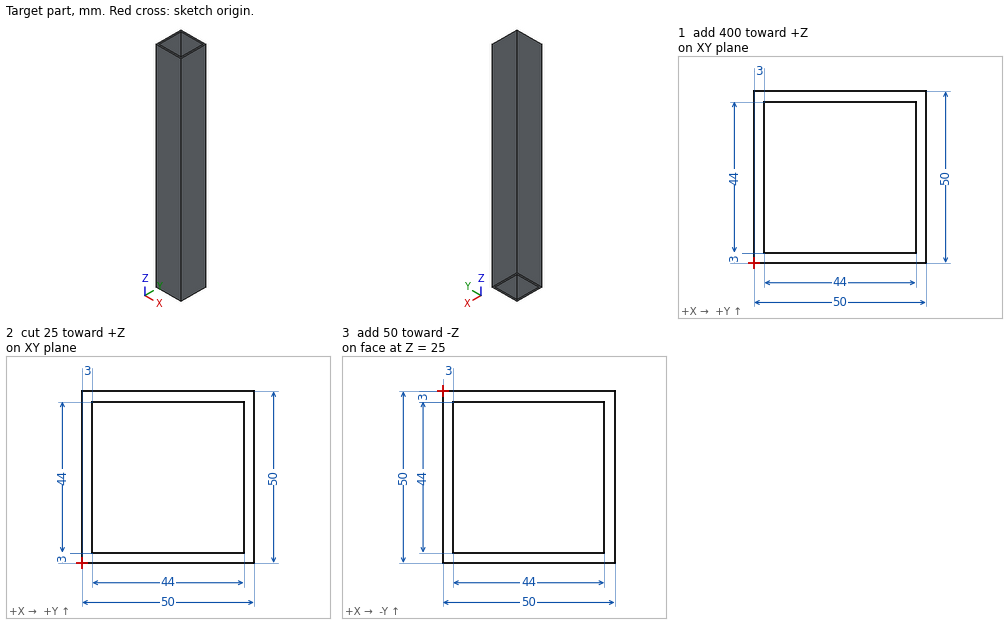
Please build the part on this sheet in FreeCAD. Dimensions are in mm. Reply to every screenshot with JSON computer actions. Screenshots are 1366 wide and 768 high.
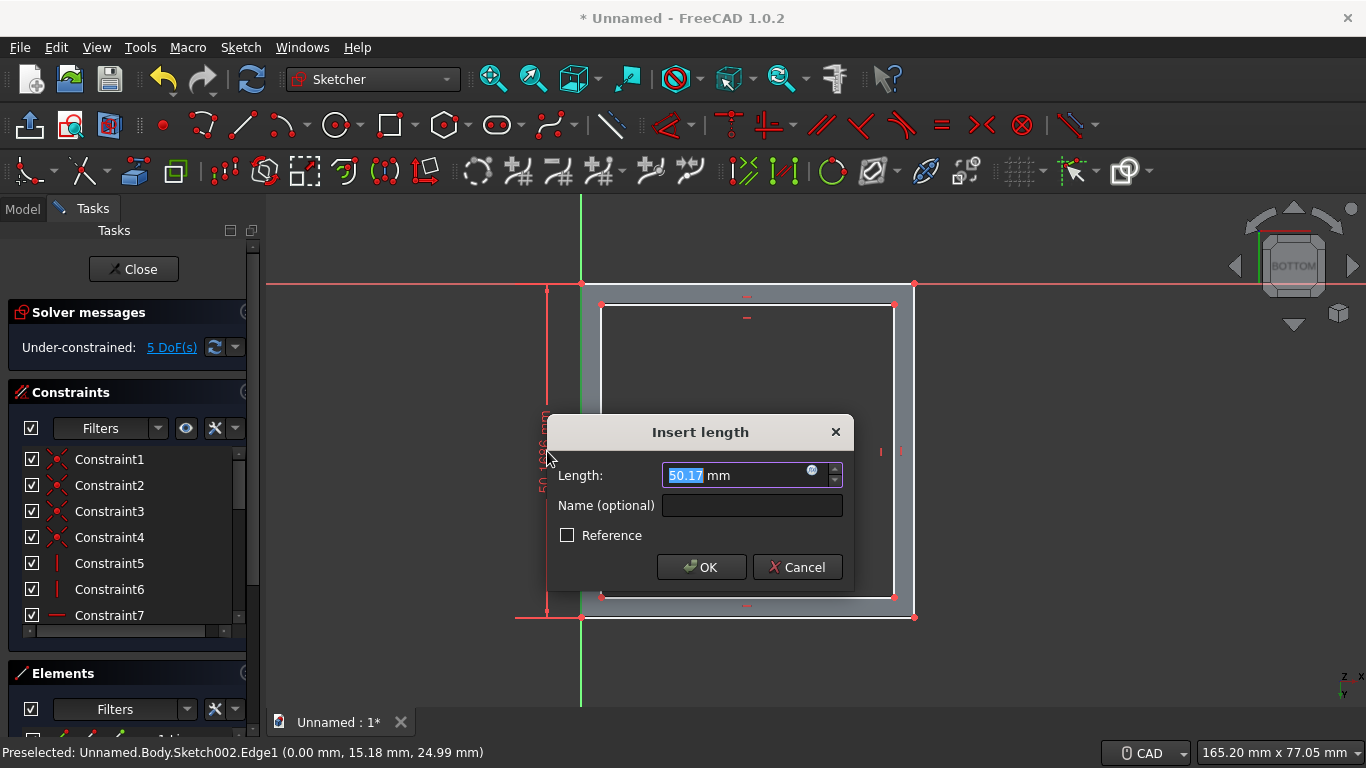
{"action": "type", "text": "50"}
{"action": "key", "text": "Return"}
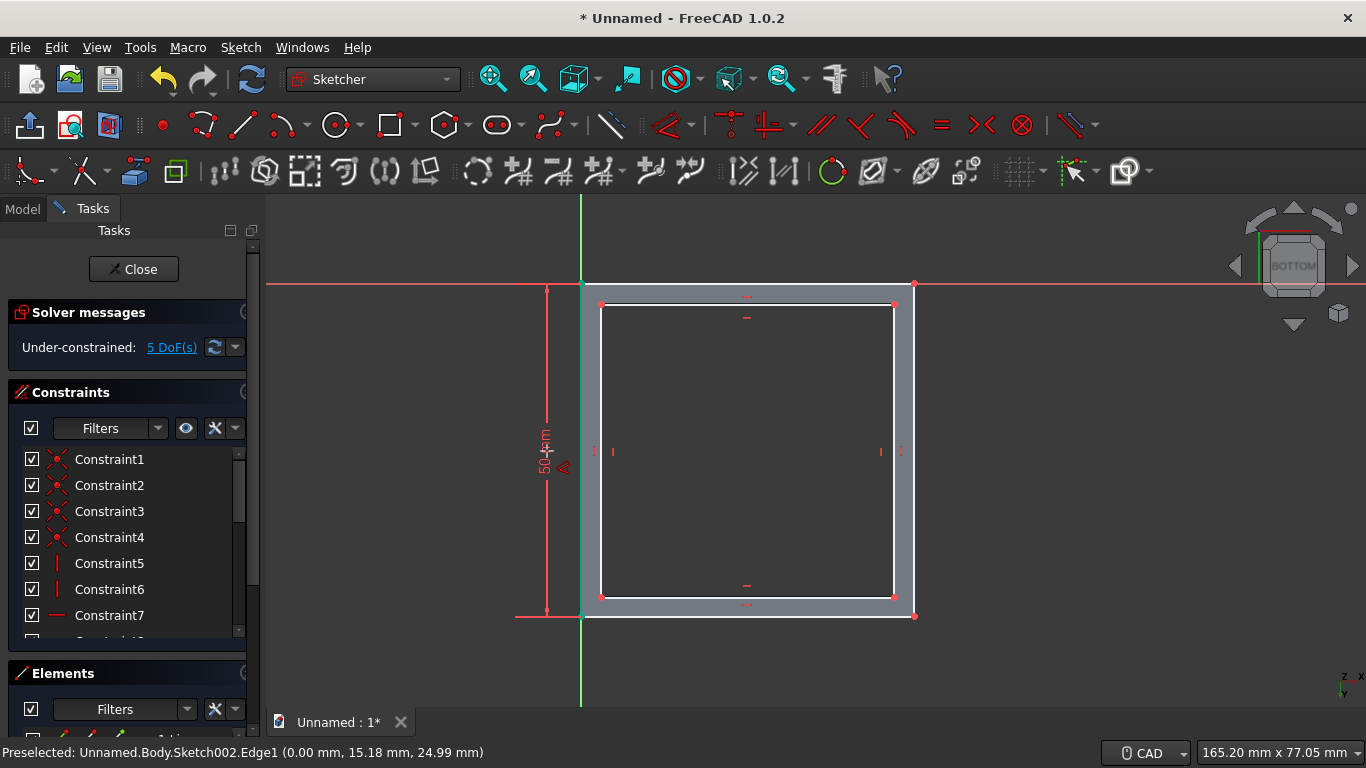
{"action": "left_click", "coordinate": [681, 617]}
{"action": "left_click", "coordinate": [748, 651]}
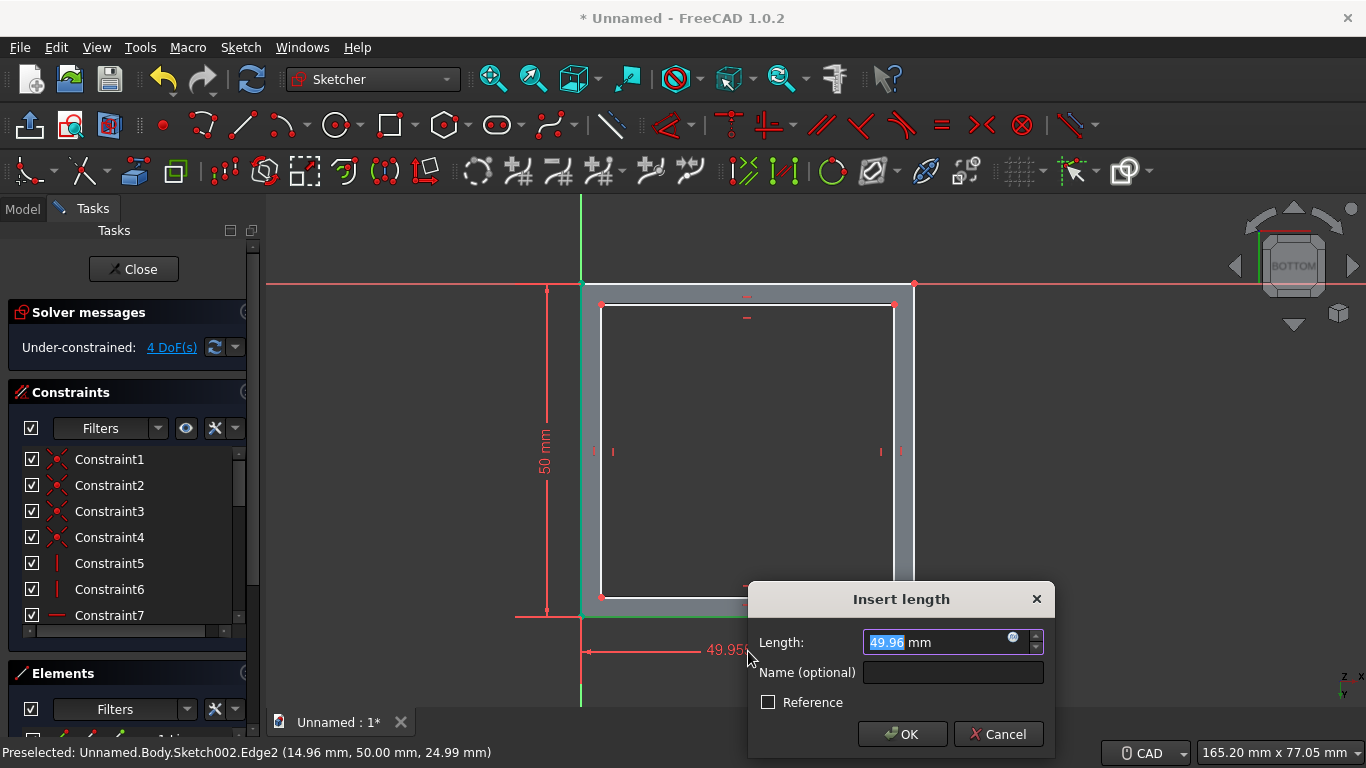
{"action": "type", "text": "50"}
{"action": "key", "text": "Return"}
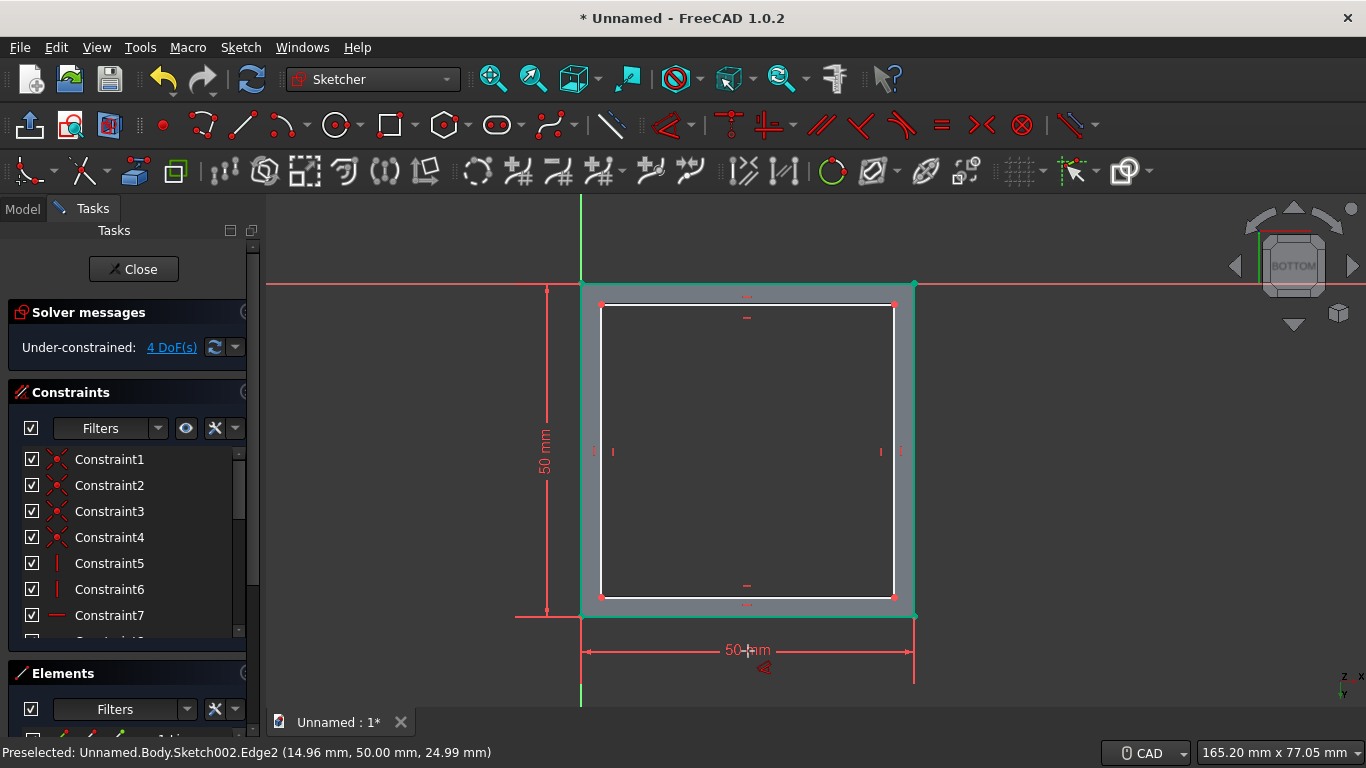
{"action": "left_click", "coordinate": [601, 393]}
{"action": "left_click", "coordinate": [567, 384]}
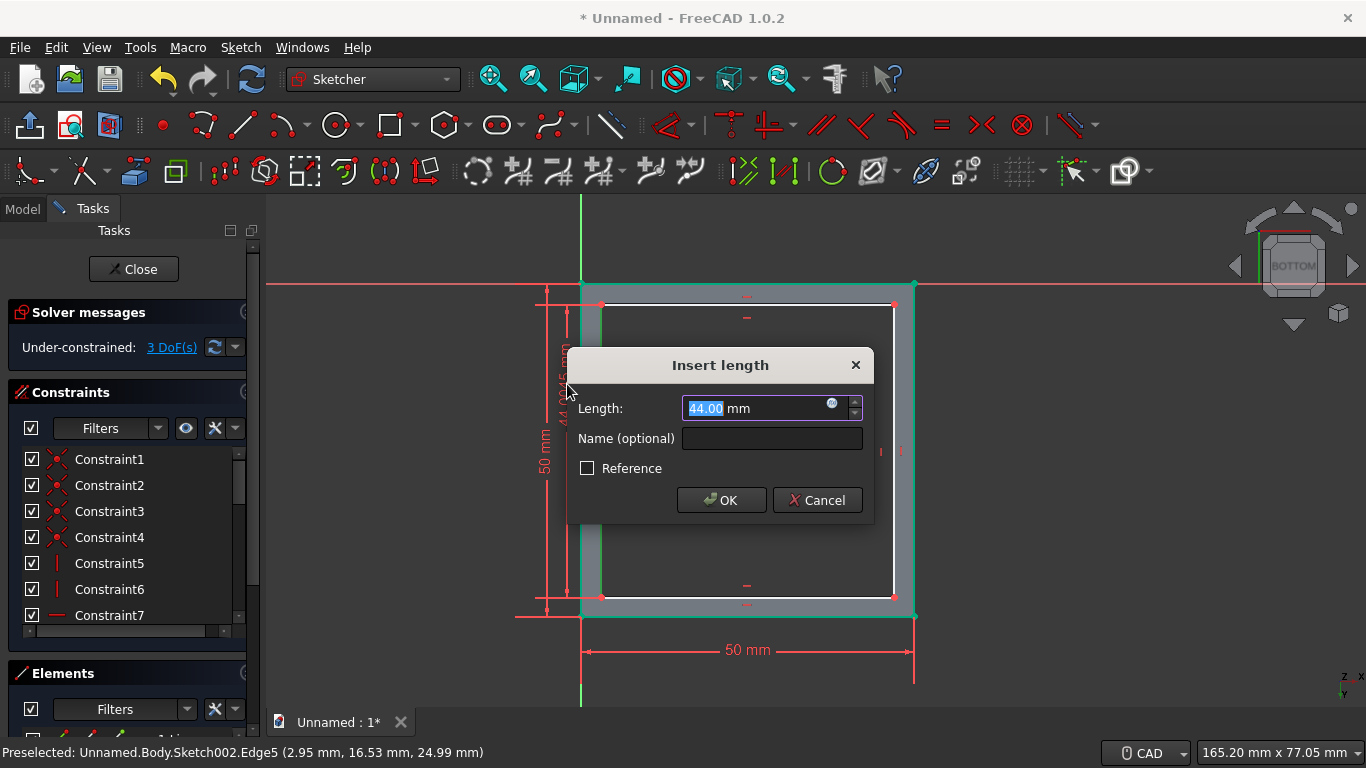
{"action": "type", "text": "44"}
{"action": "key", "text": "Return"}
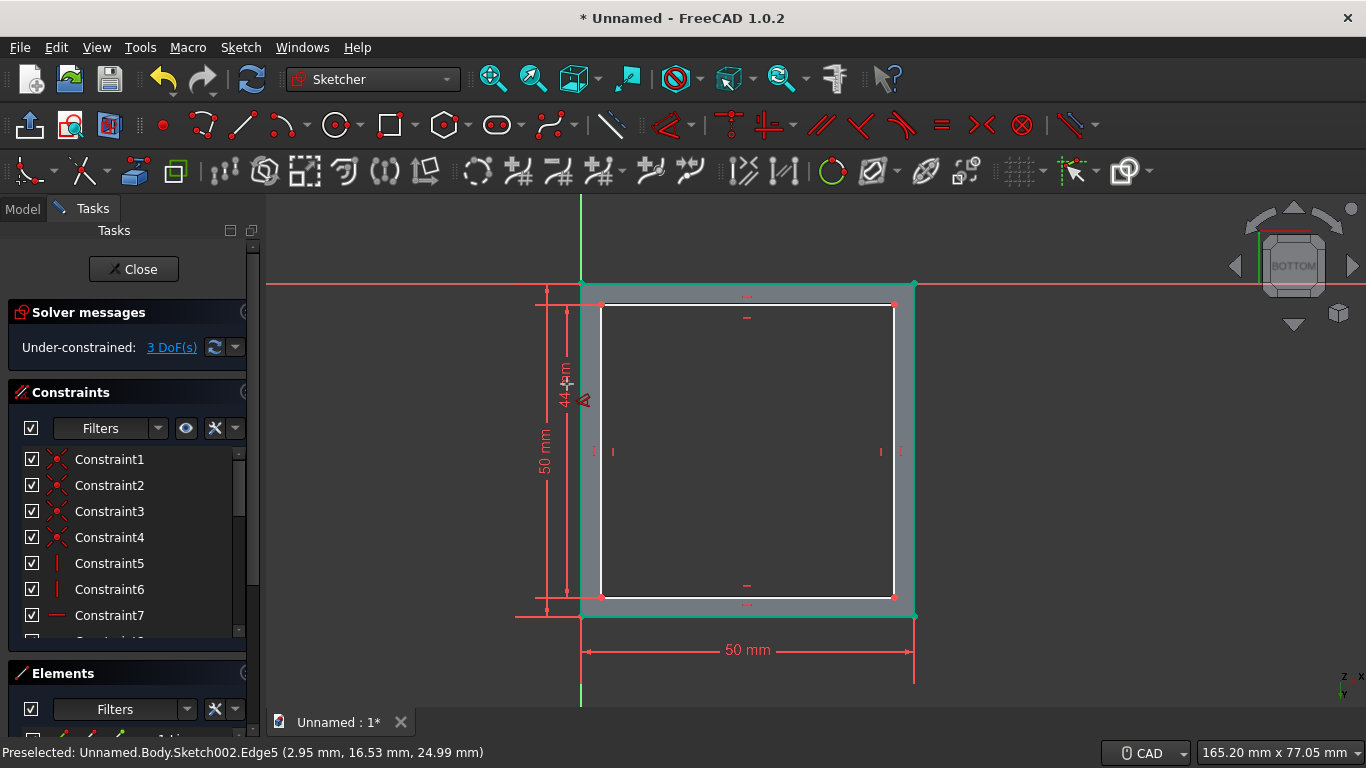
{"action": "left_click", "coordinate": [689, 598]}
{"action": "left_click", "coordinate": [645, 632]}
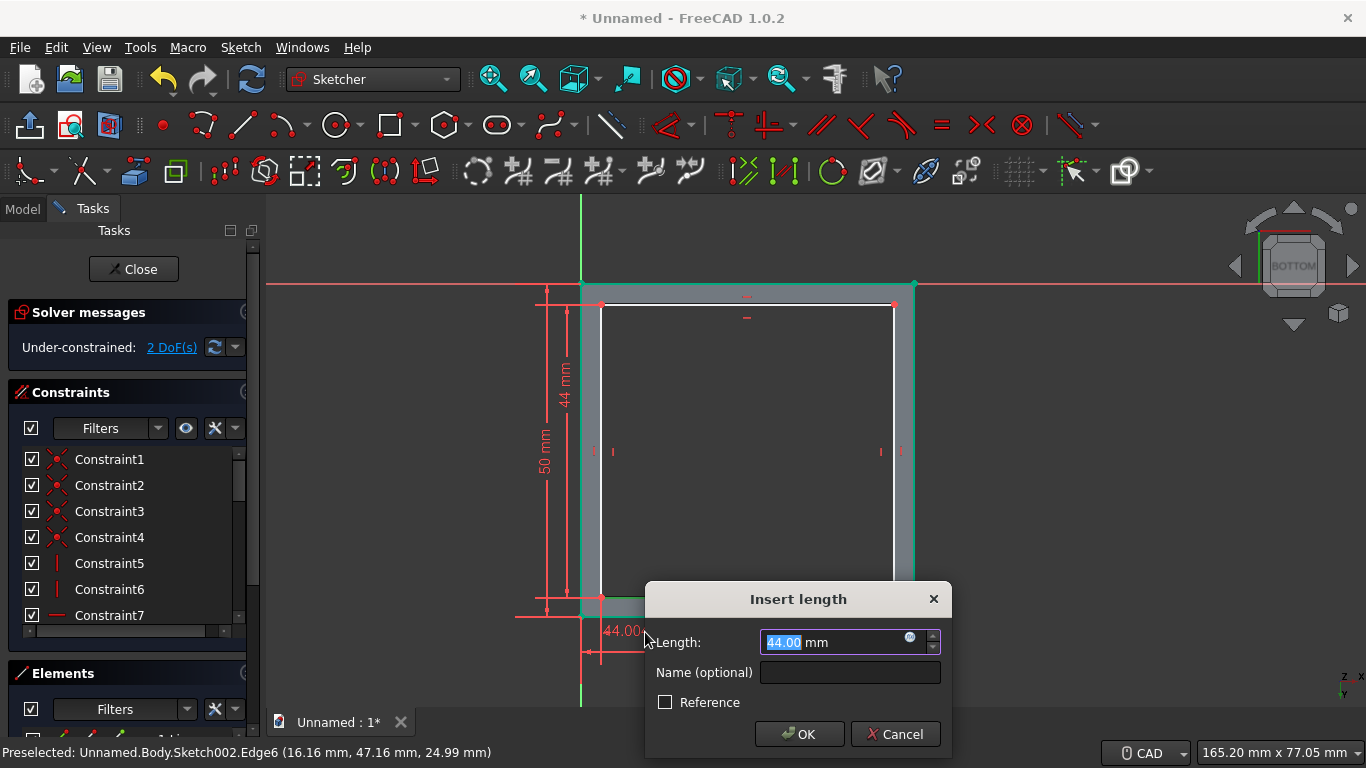
{"action": "type", "text": "44"}
{"action": "key", "text": "Return"}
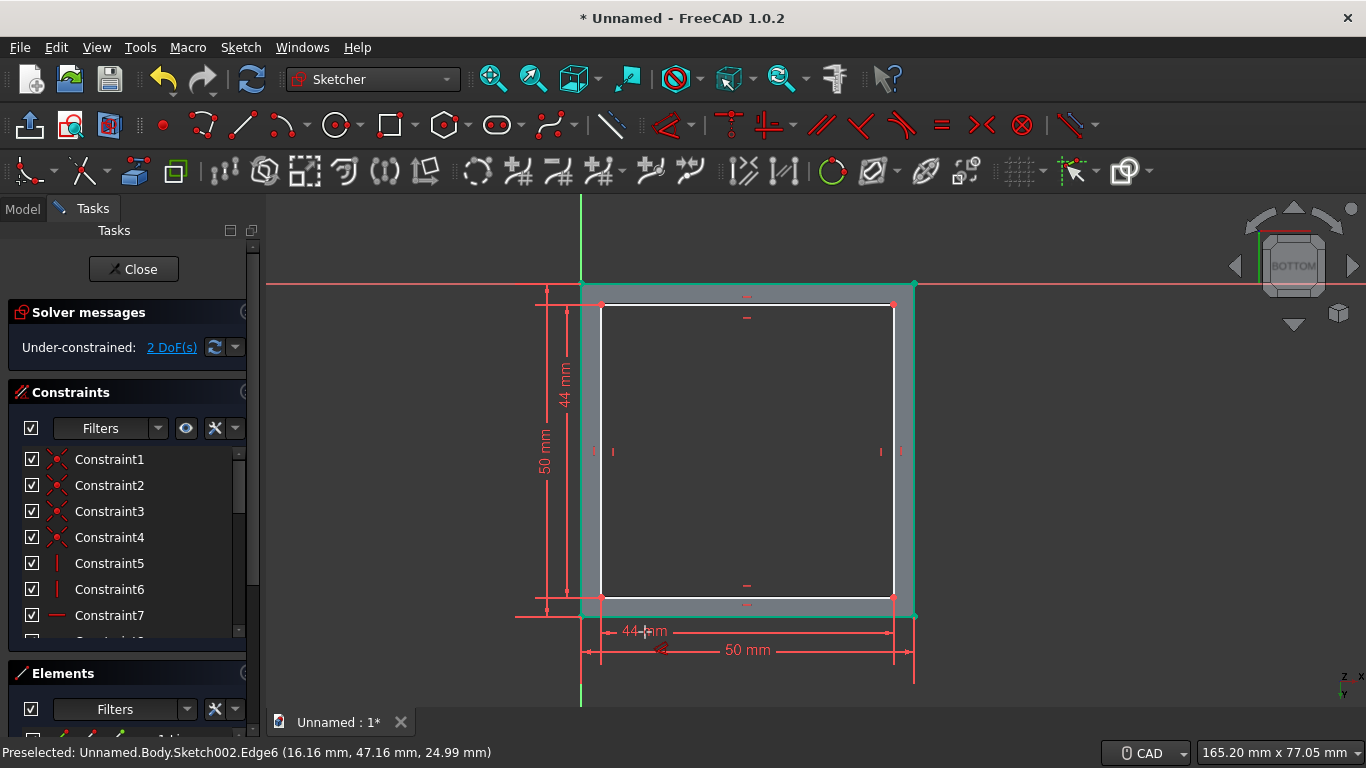
{"action": "scroll", "coordinate": [601, 305], "scroll_direction": "up", "scroll_amount": 4}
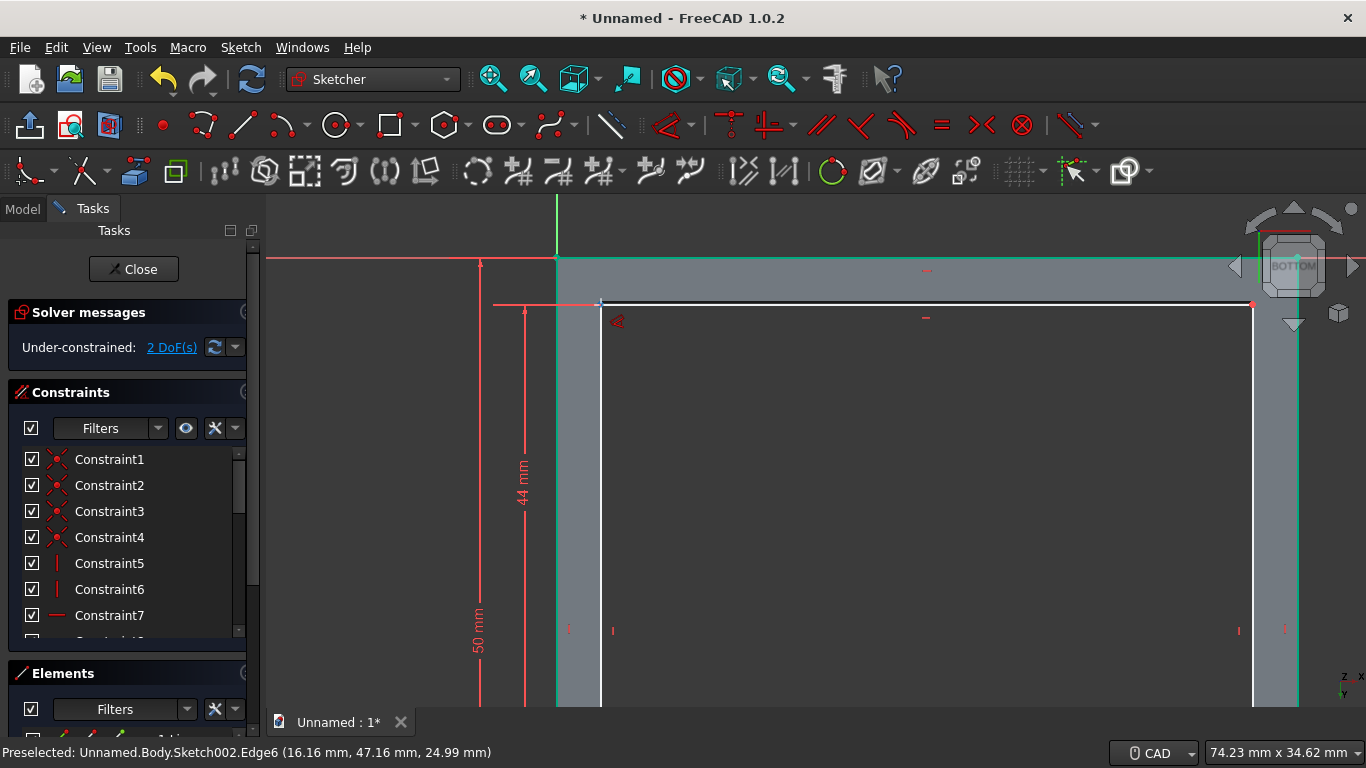
{"action": "left_click", "coordinate": [601, 305]}
{"action": "left_click", "coordinate": [579, 224]}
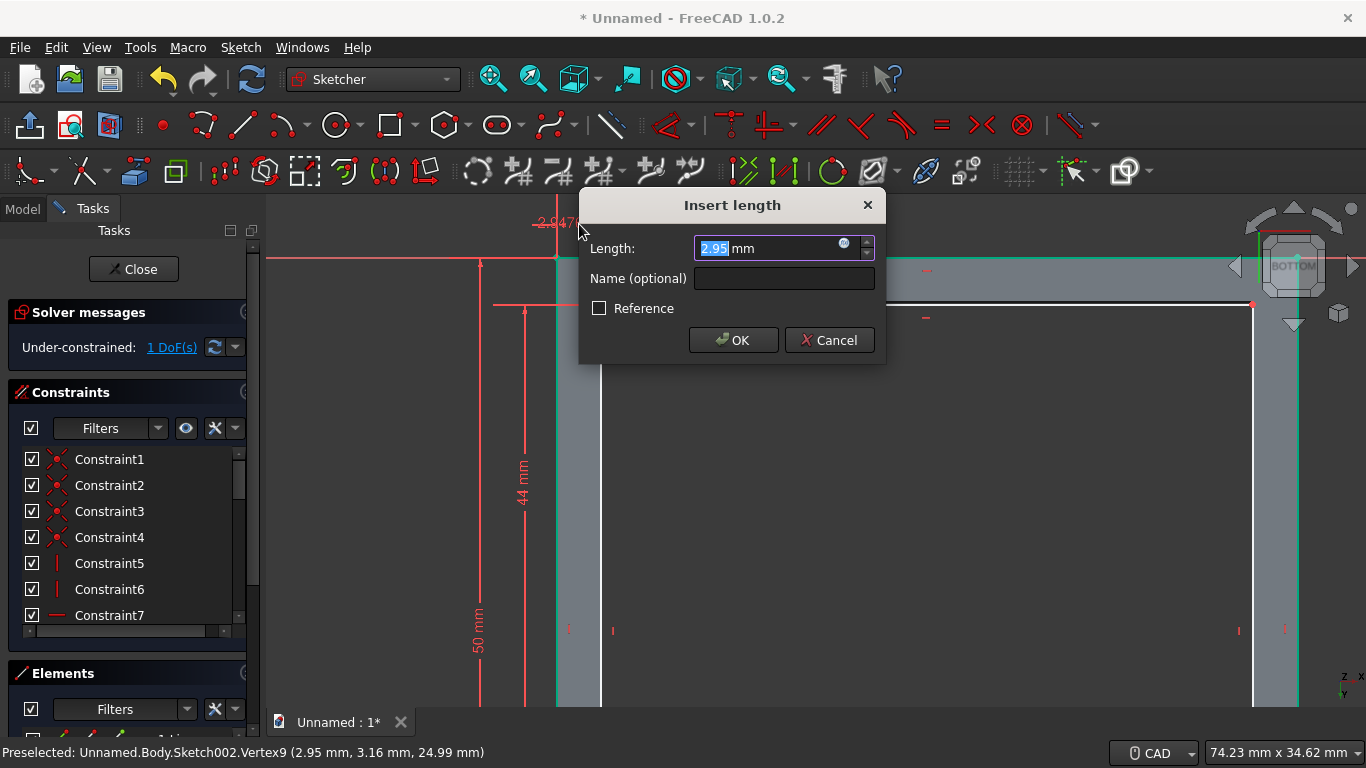
{"action": "type", "text": "3"}
{"action": "key", "text": "Return"}